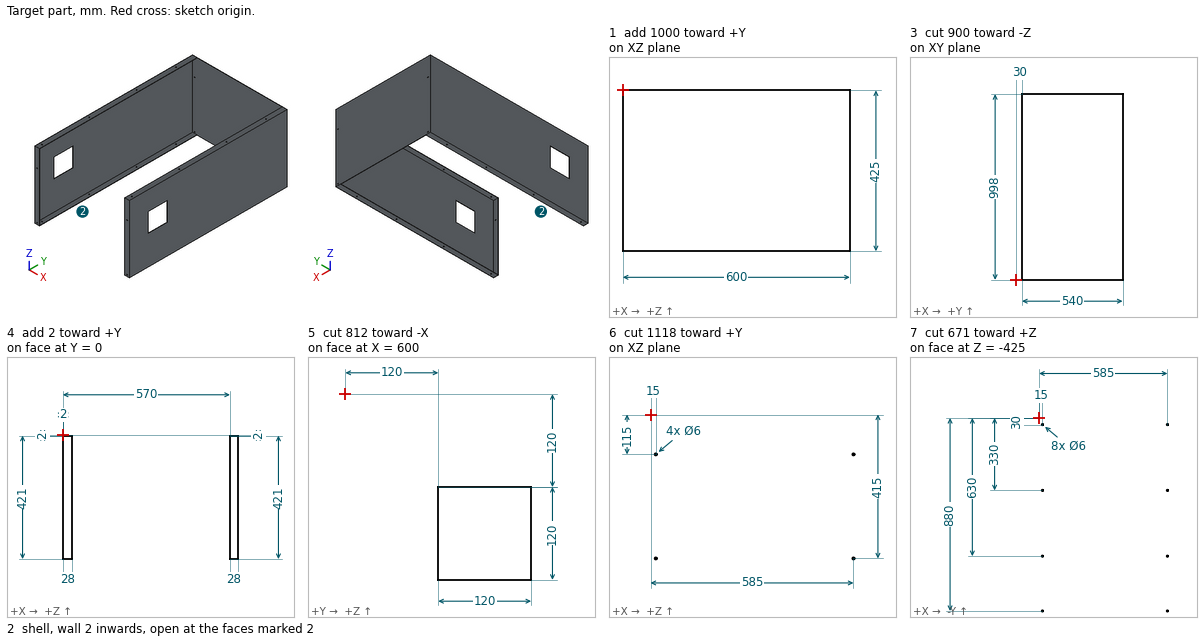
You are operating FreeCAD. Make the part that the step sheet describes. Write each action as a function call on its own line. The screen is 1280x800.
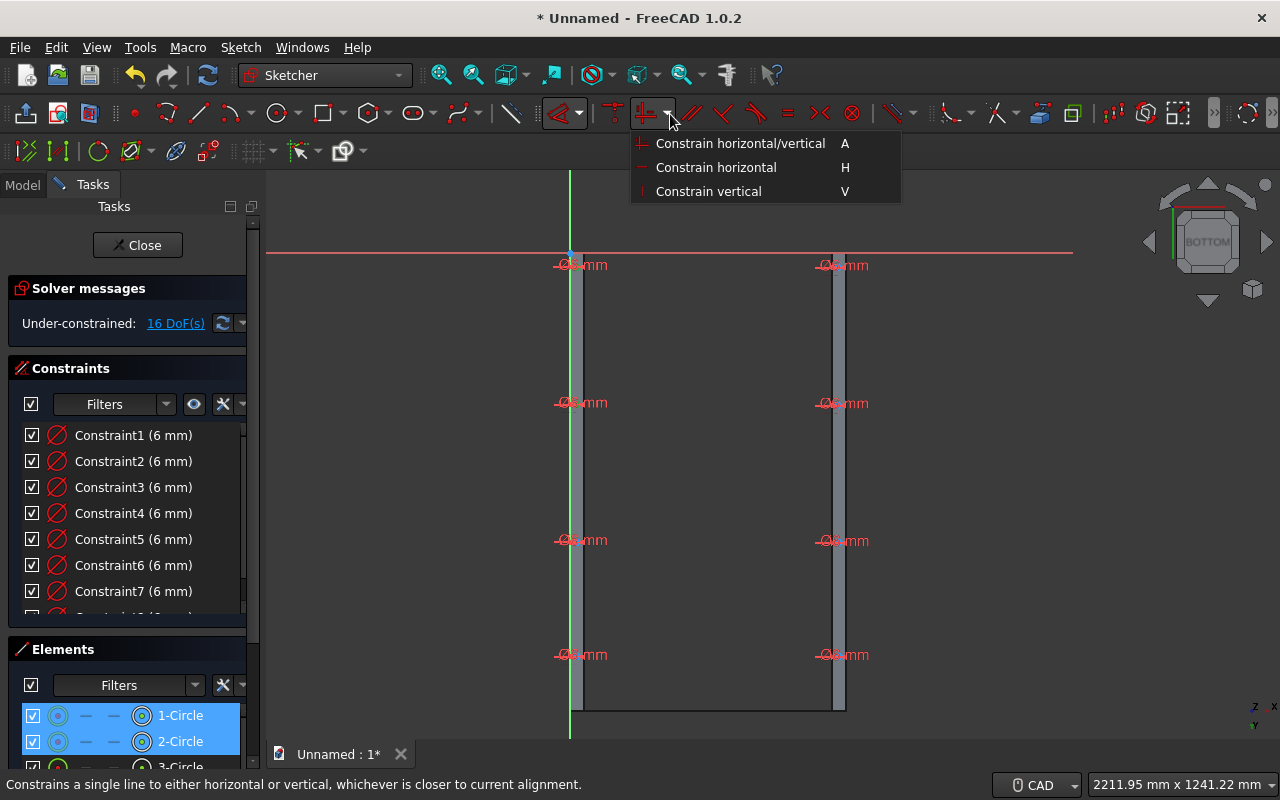
click(766, 191)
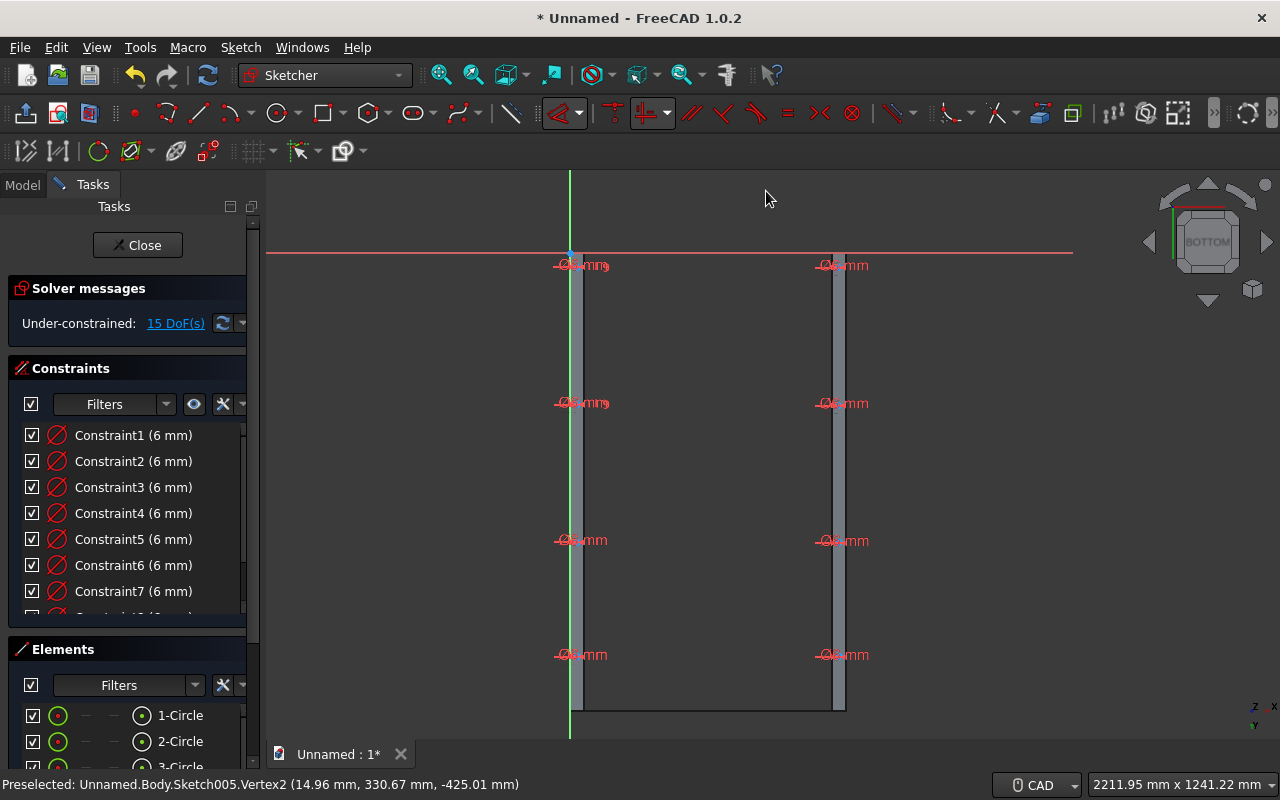
click(577, 405)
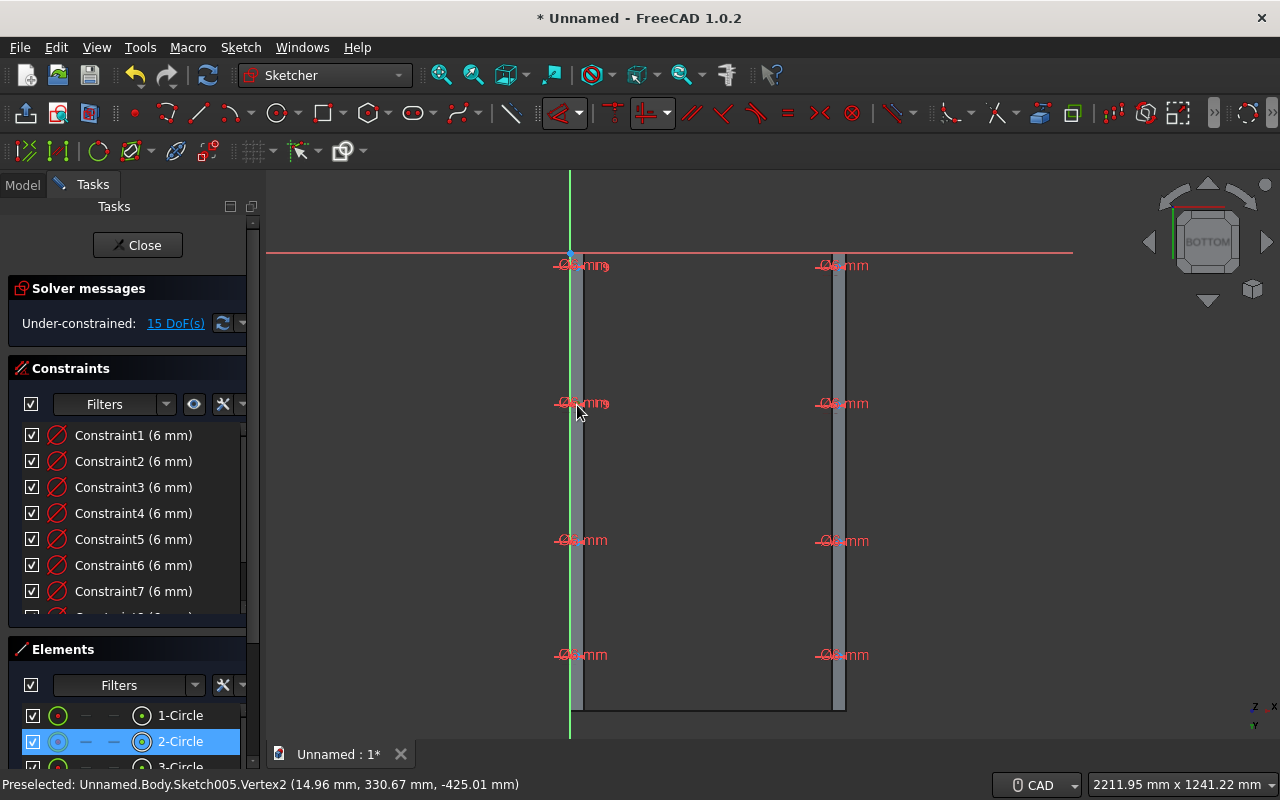
click(577, 542)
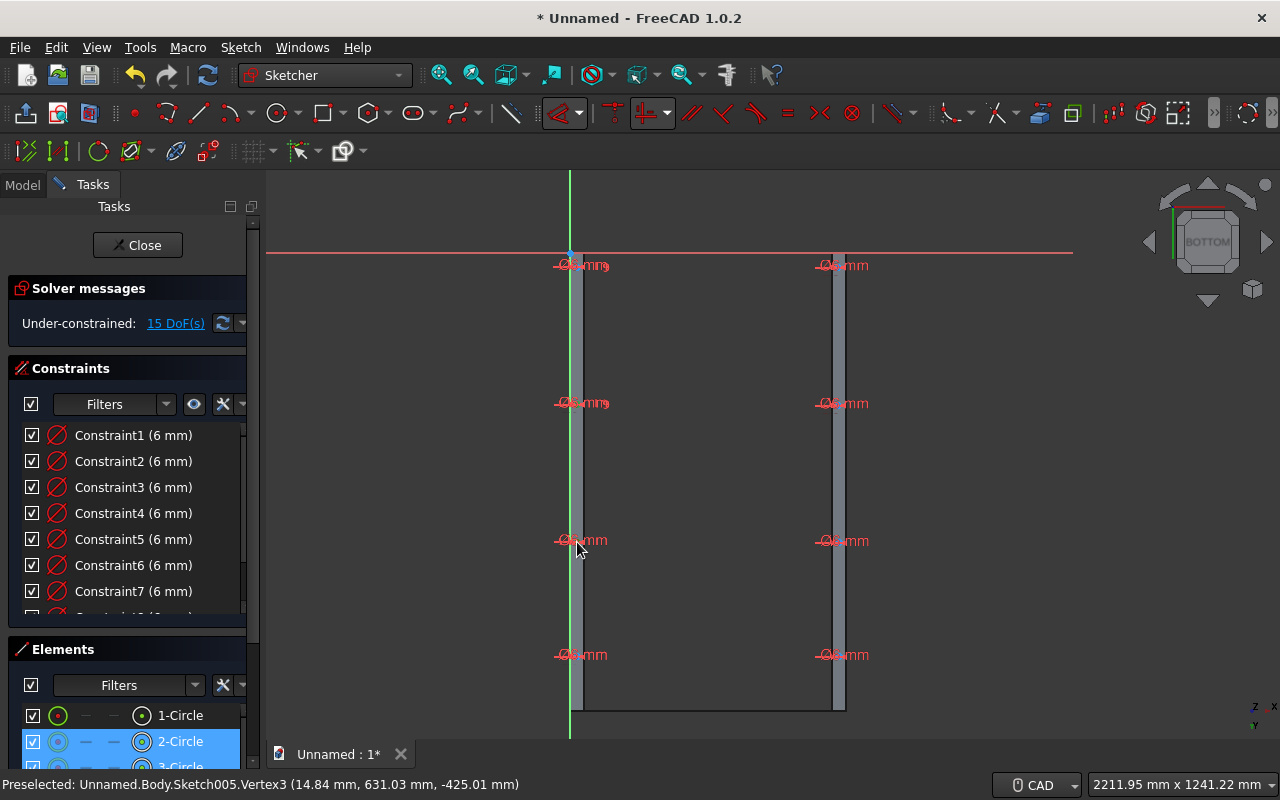
click(670, 114)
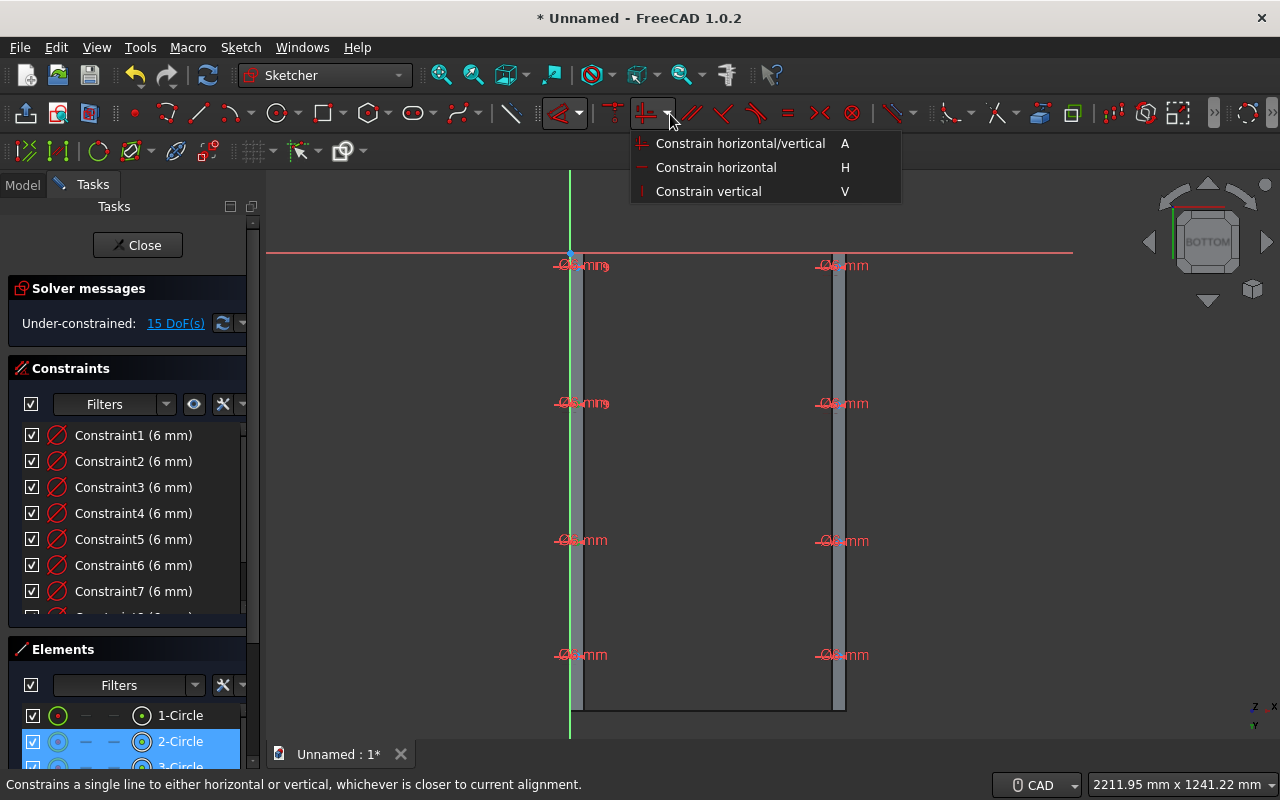
click(766, 191)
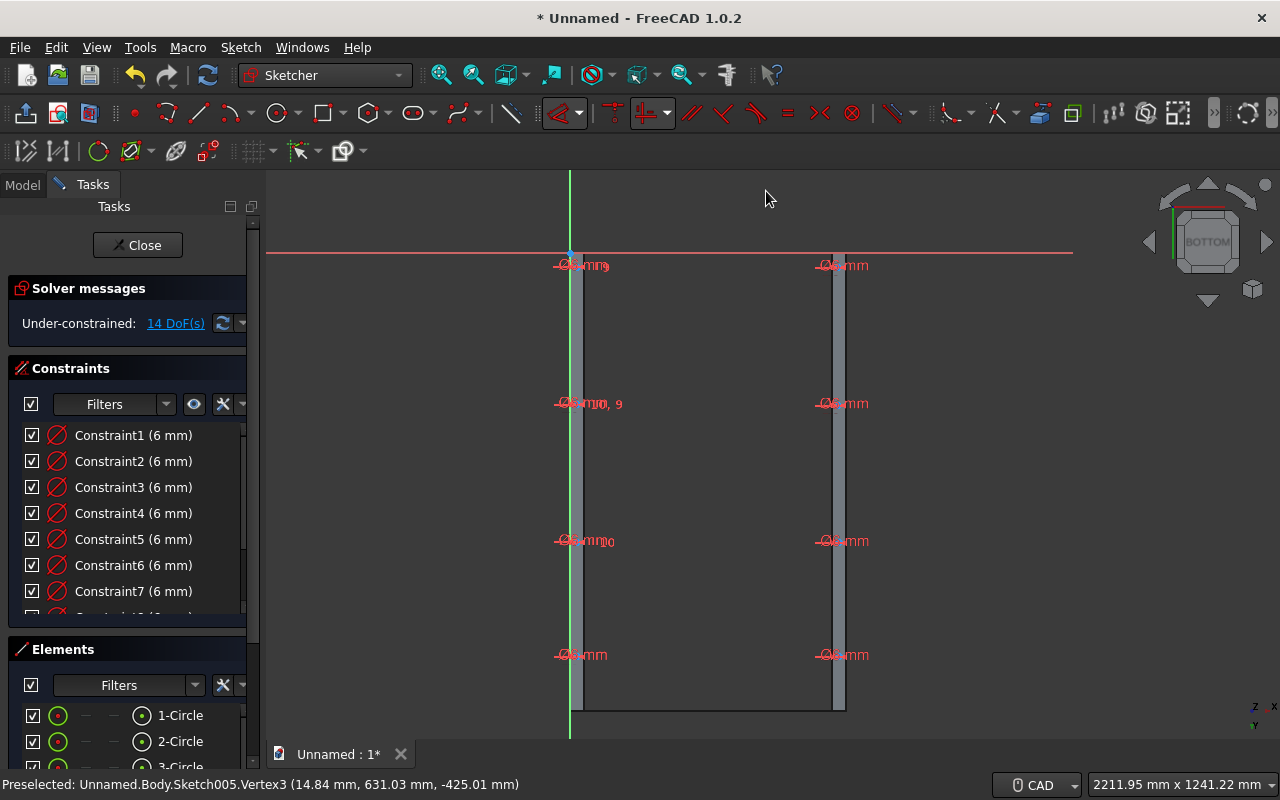
click(577, 267)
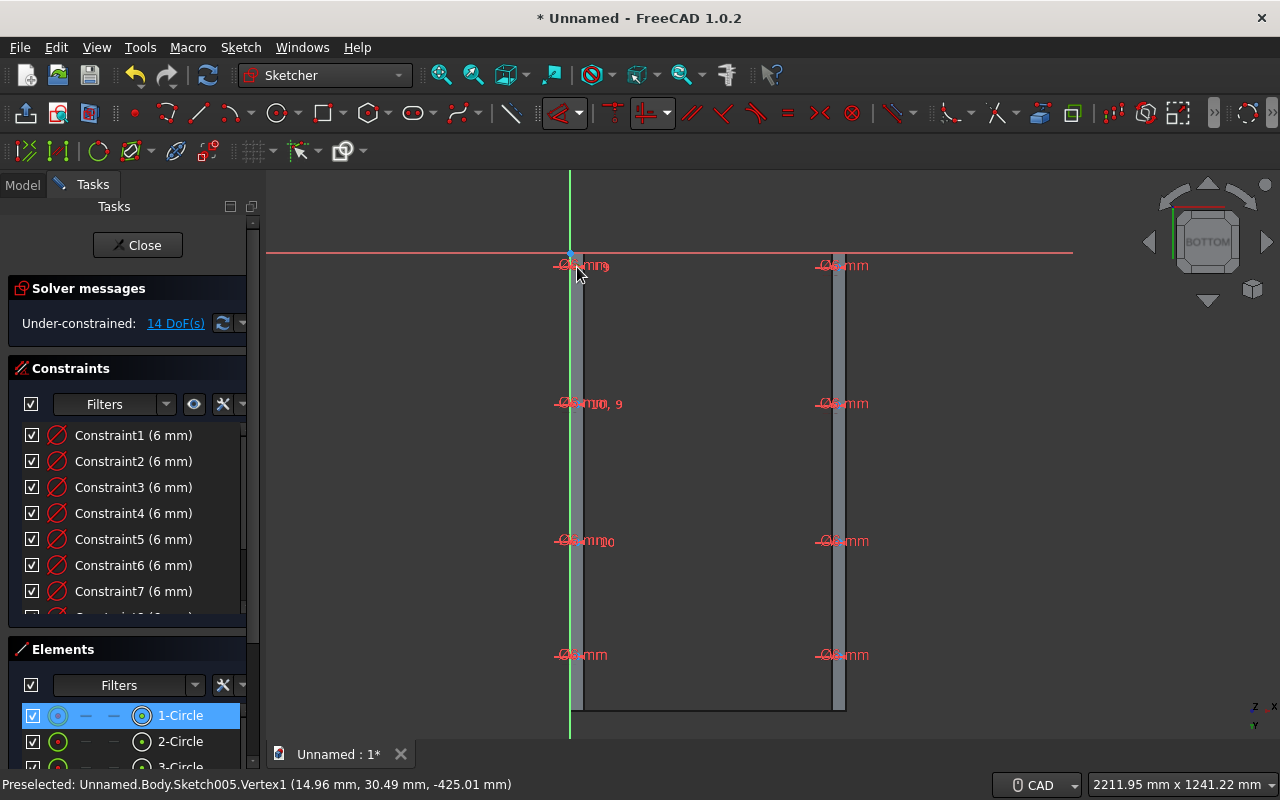
click(838, 268)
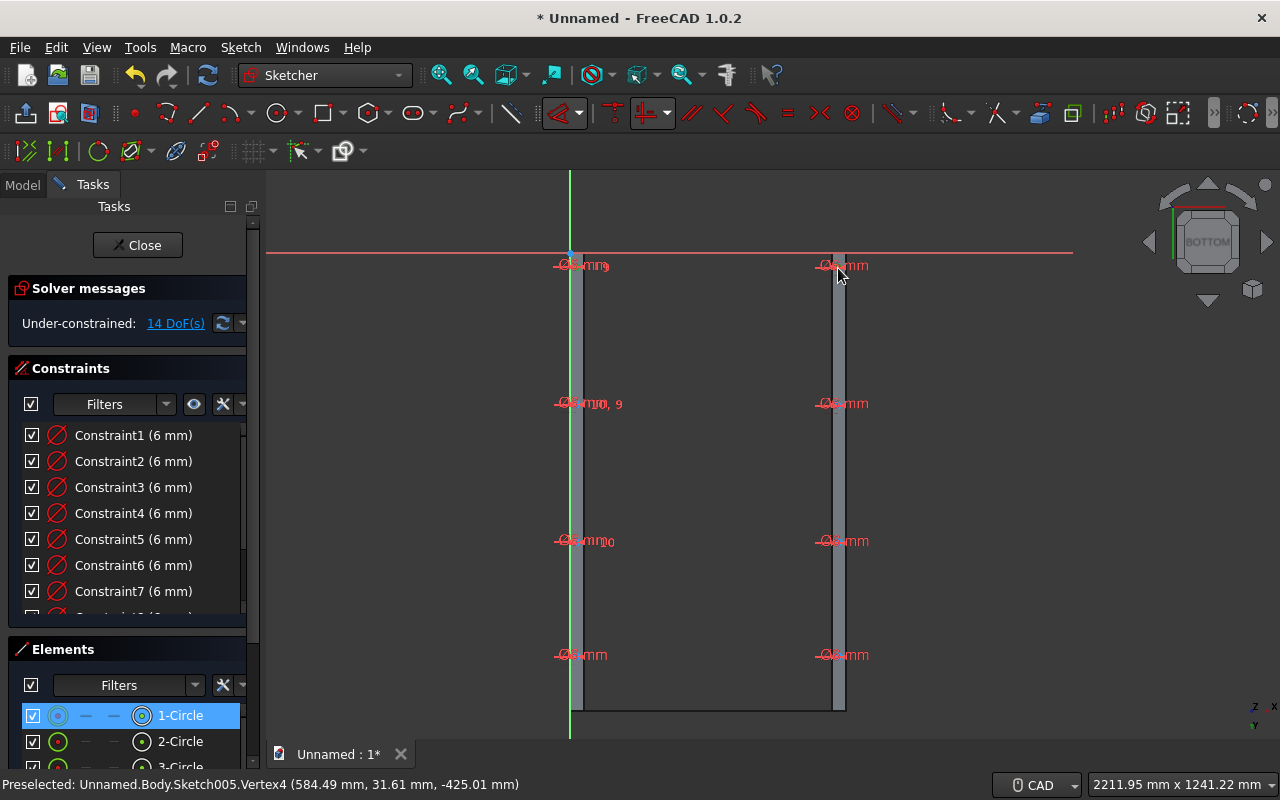
click(670, 114)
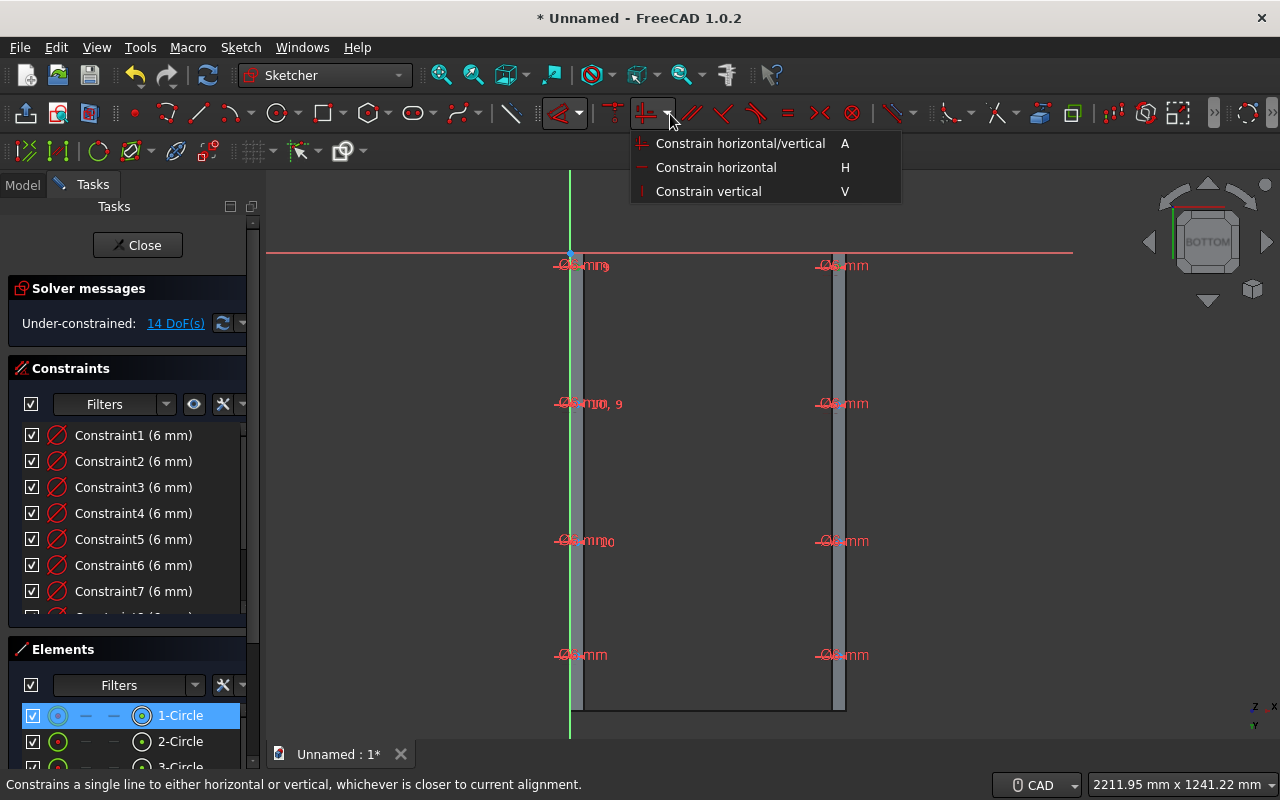
click(766, 167)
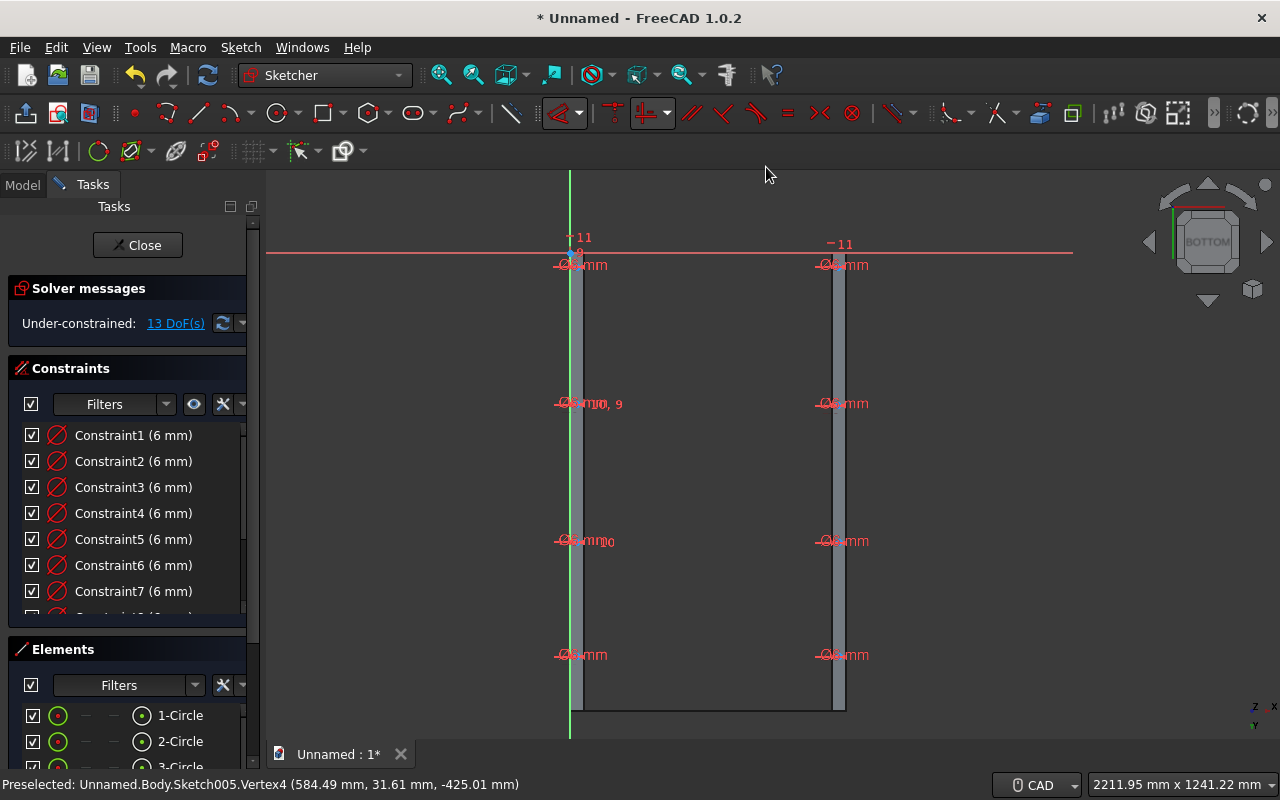
click(838, 267)